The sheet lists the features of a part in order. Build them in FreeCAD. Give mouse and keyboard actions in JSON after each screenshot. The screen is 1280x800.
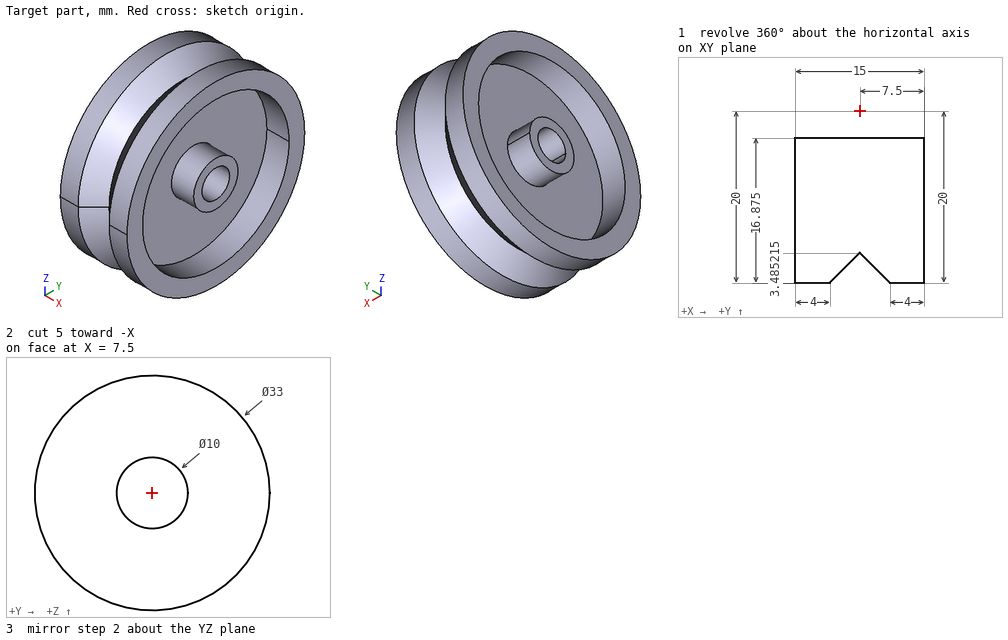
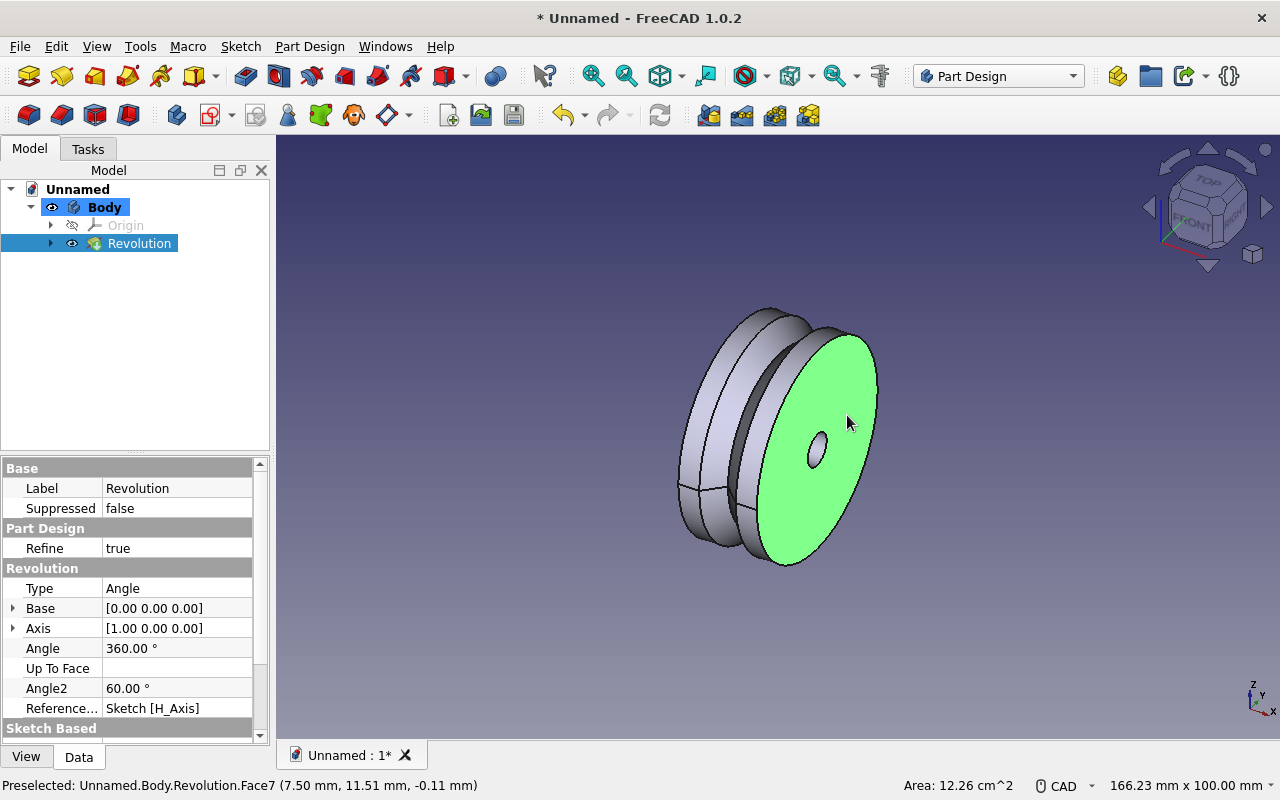
{"action": "left_click", "coordinate": [210, 116]}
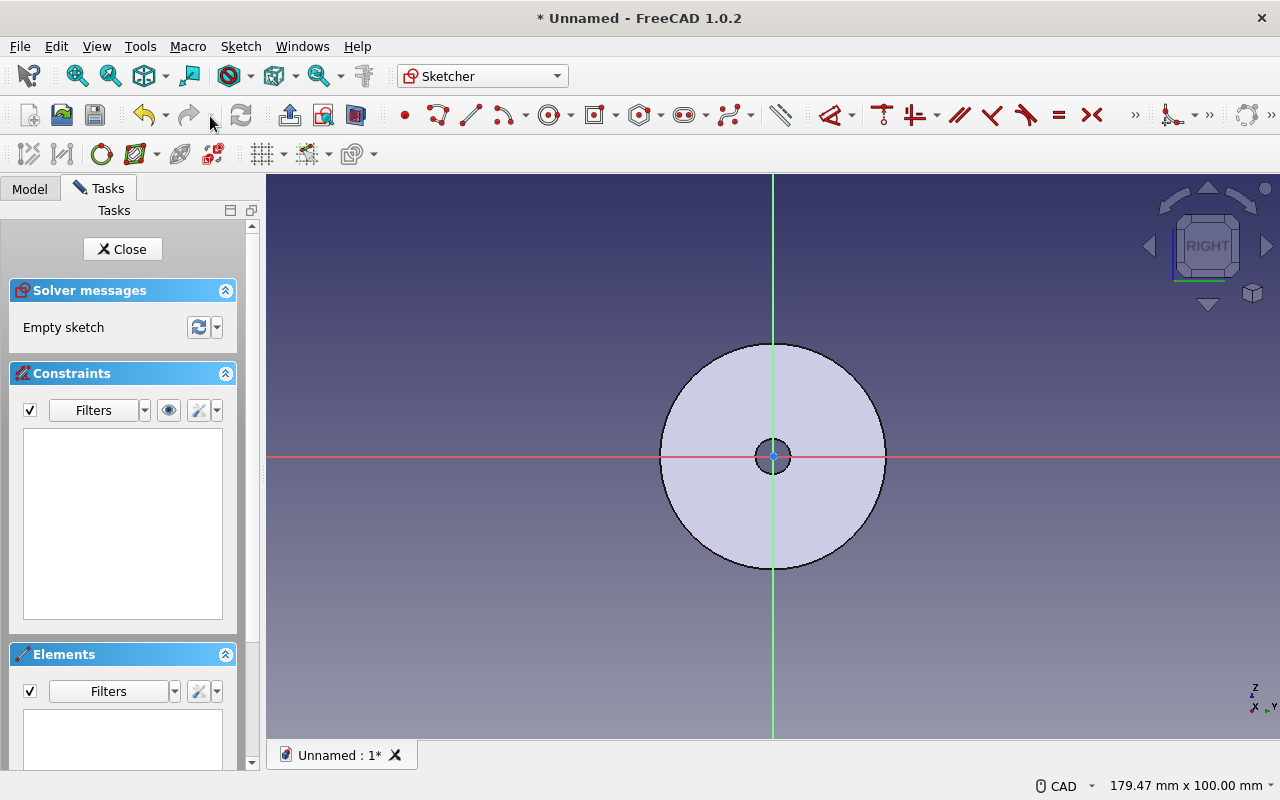
{"action": "scroll", "coordinate": [856, 456], "scroll_direction": "up", "scroll_amount": 3}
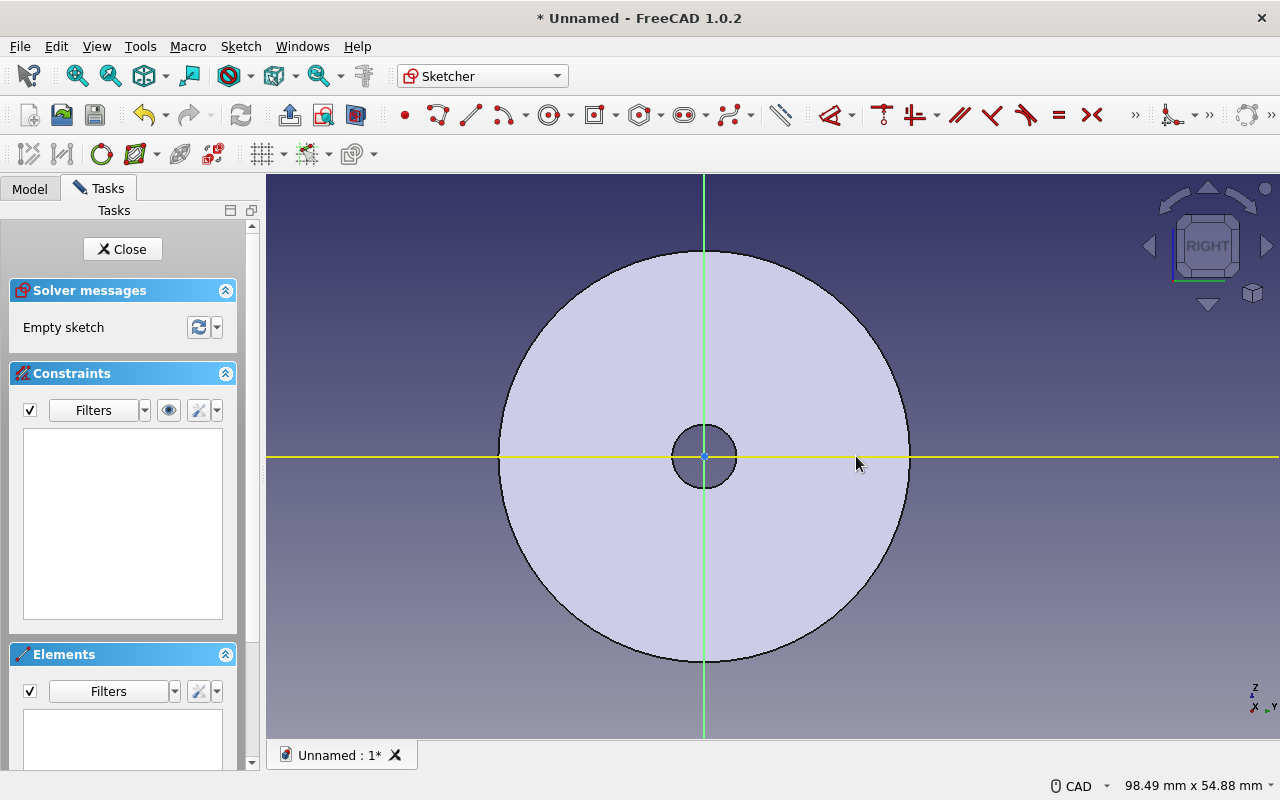
{"action": "left_click", "coordinate": [548, 116]}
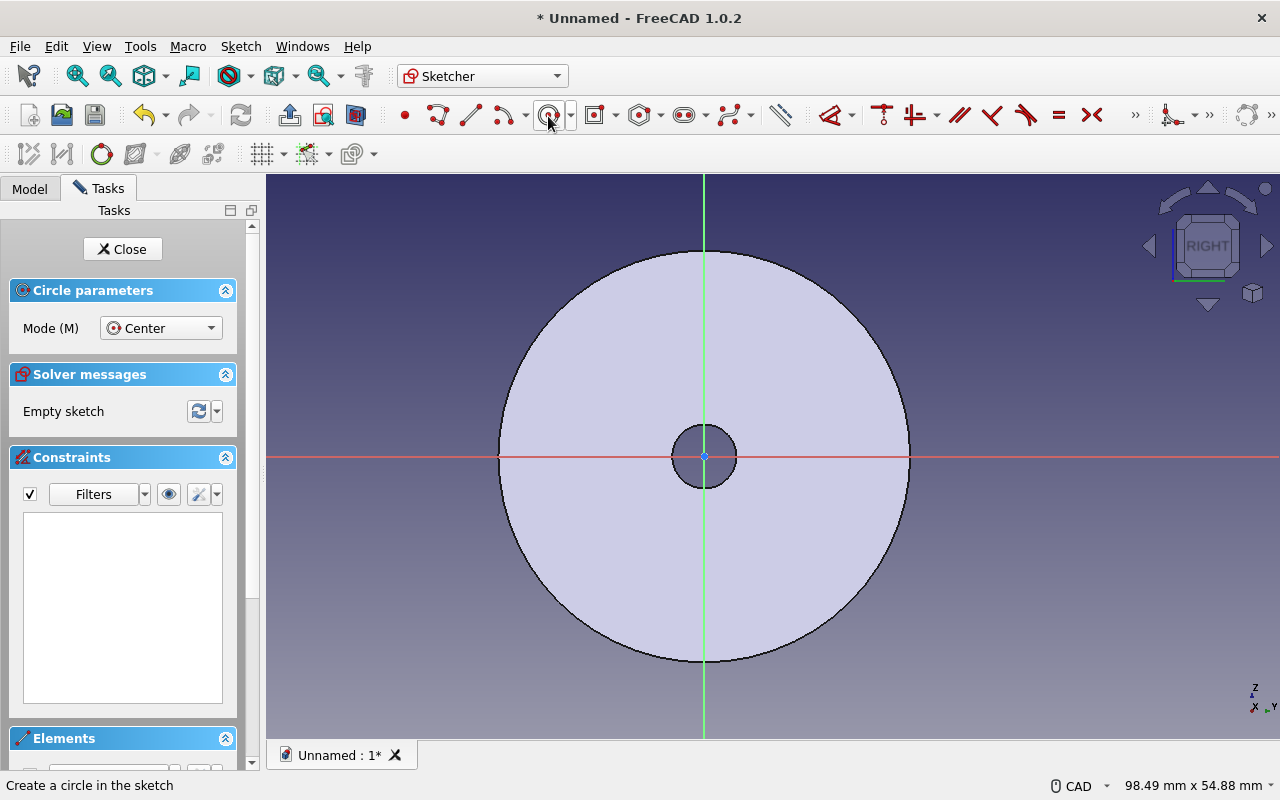
{"action": "left_click", "coordinate": [704, 456]}
{"action": "mouse_move", "coordinate": [824, 336]}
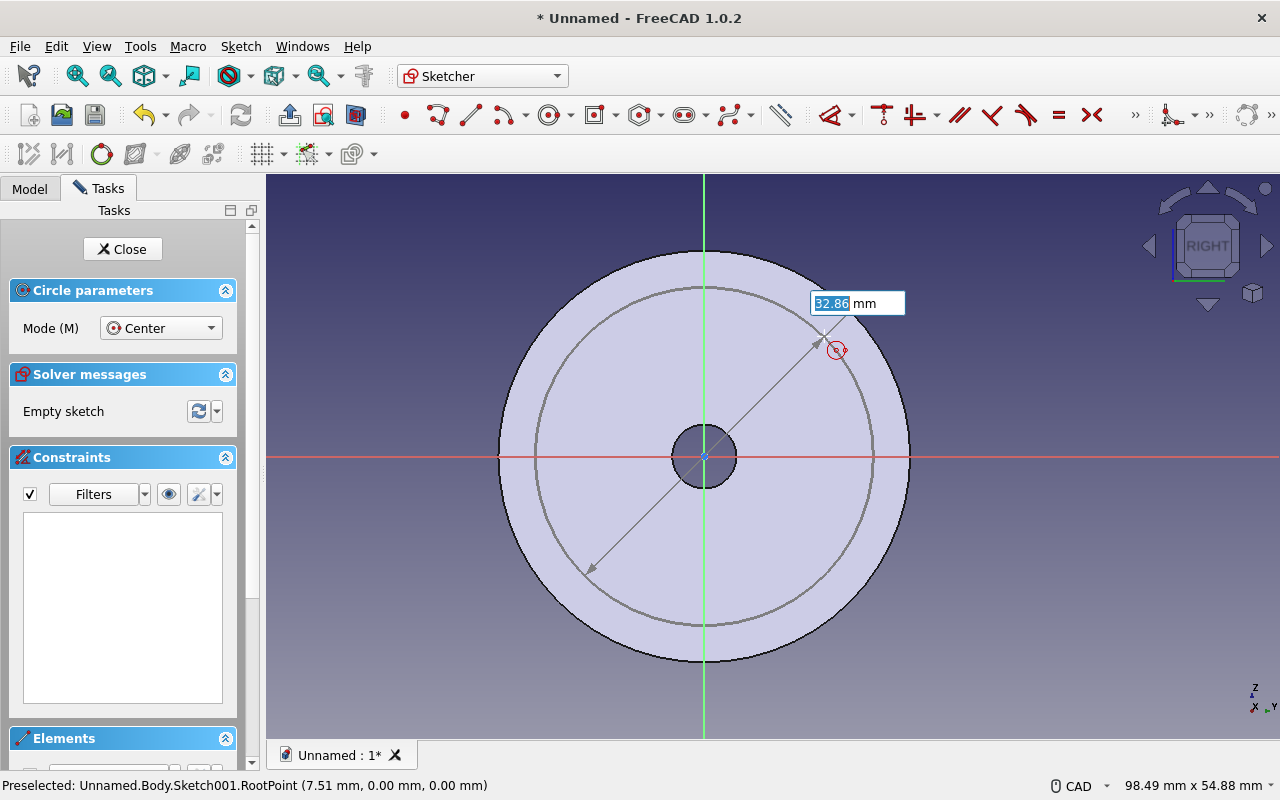
{"action": "type", "text": "33"}
{"action": "key", "text": "Return"}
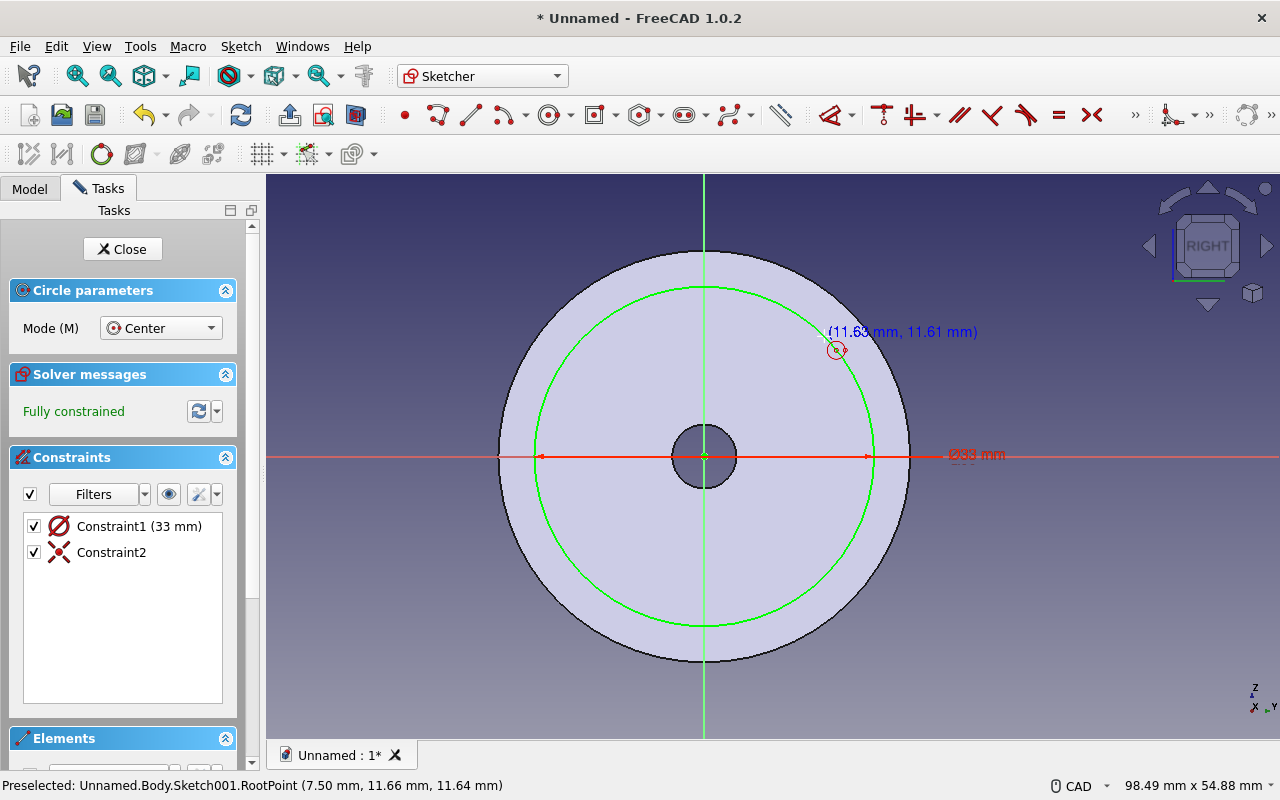
{"action": "left_click", "coordinate": [704, 456]}
{"action": "mouse_move", "coordinate": [741, 420]}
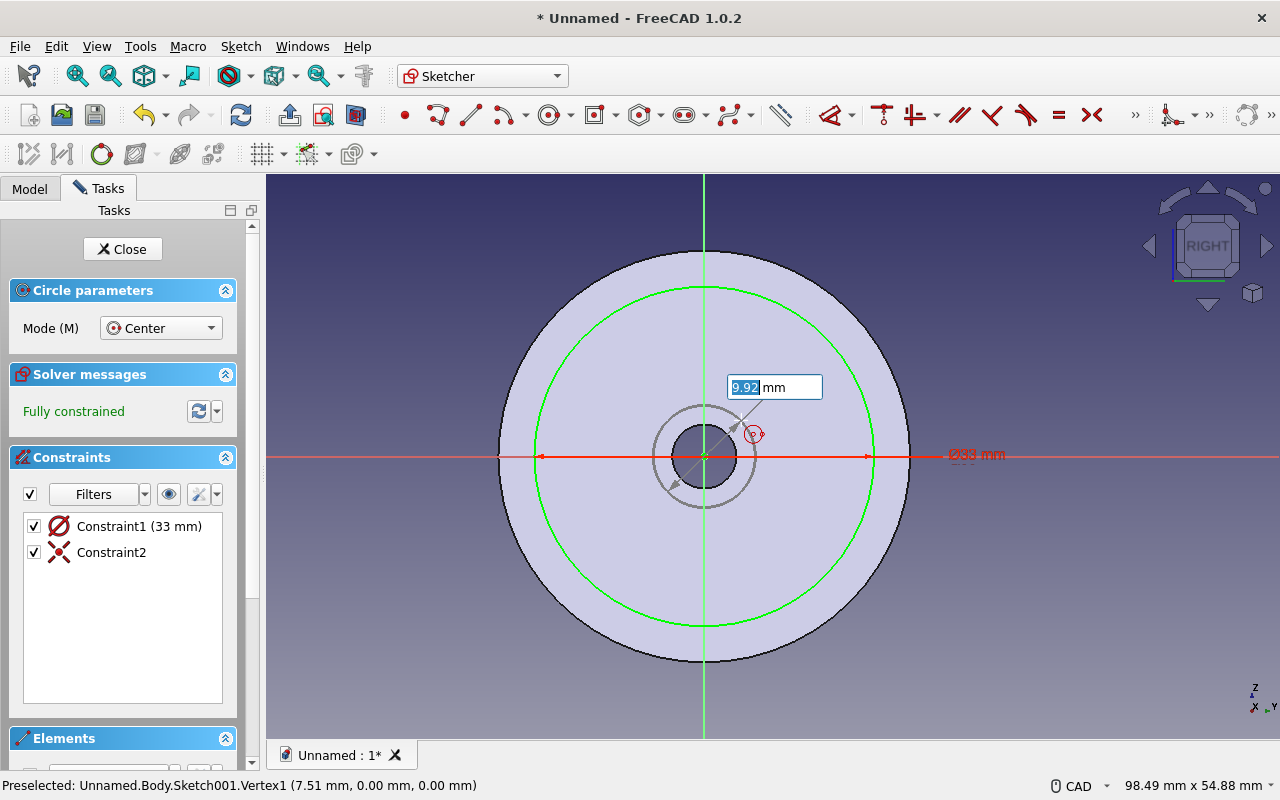
{"action": "type", "text": "10"}
{"action": "key", "text": "Return"}
{"action": "key", "text": "Escape"}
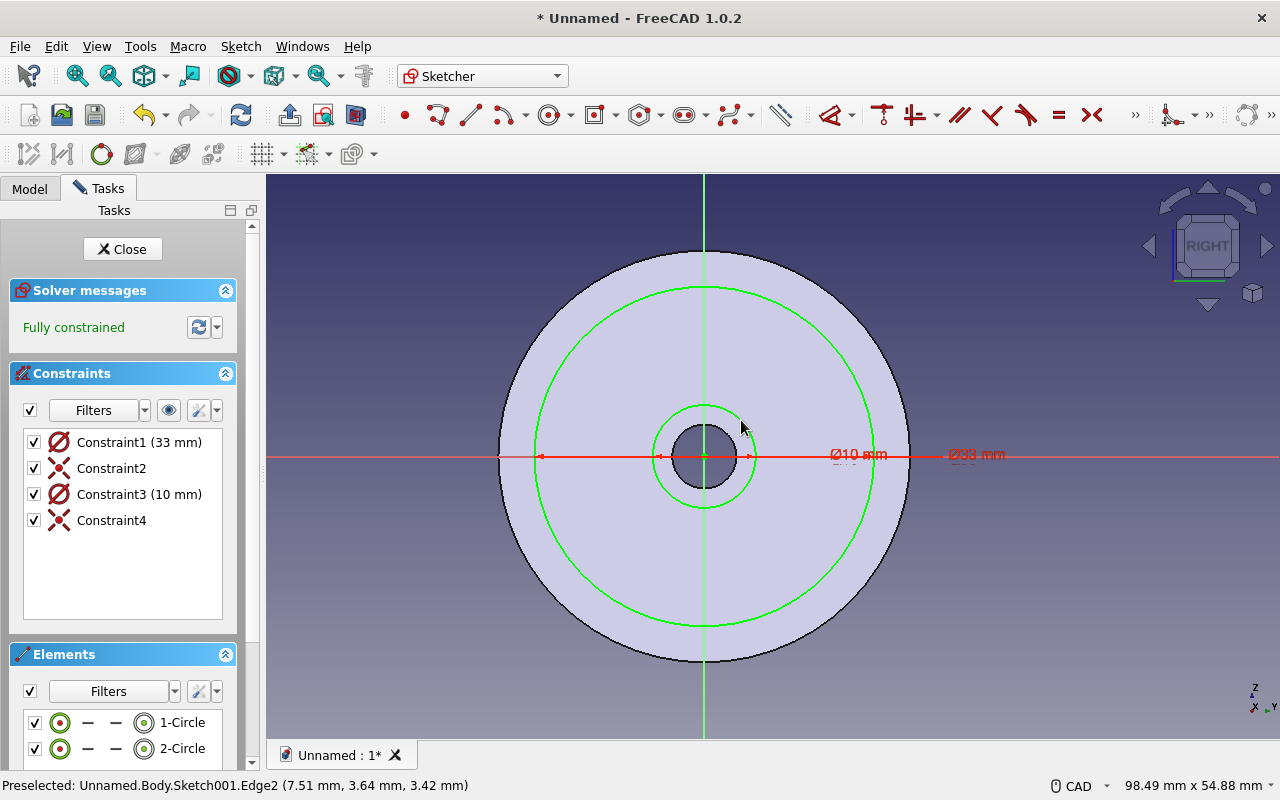
{"action": "left_click", "coordinate": [123, 249]}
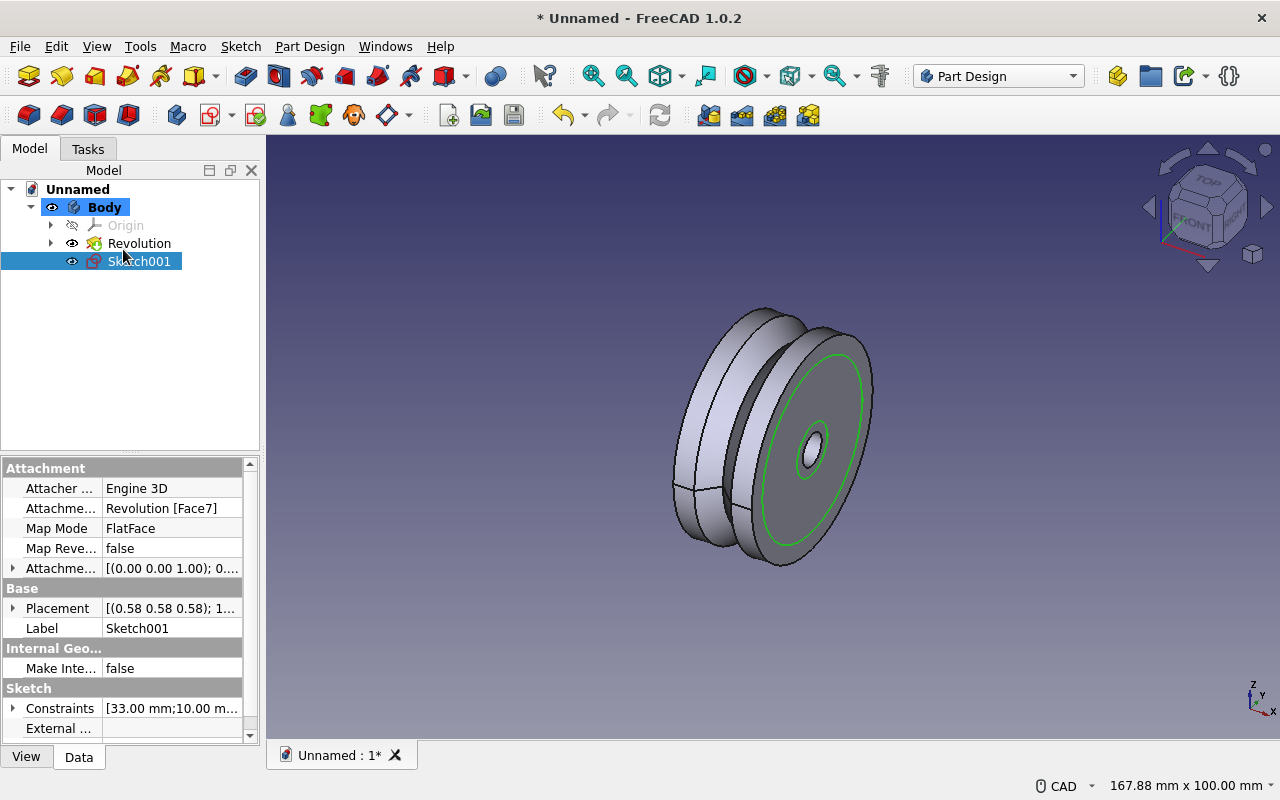
{"action": "left_click", "coordinate": [246, 76]}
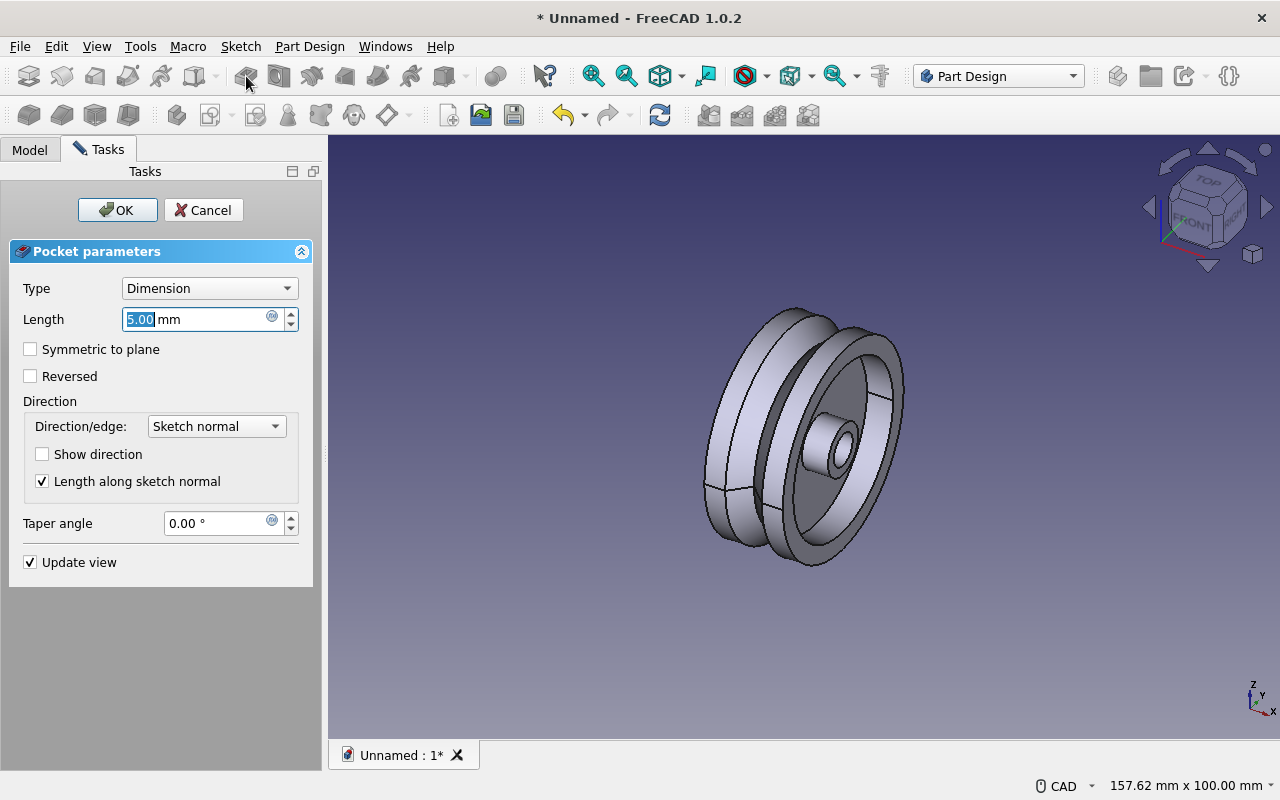
{"action": "type", "text": "5"}
{"action": "key", "text": "Tab"}